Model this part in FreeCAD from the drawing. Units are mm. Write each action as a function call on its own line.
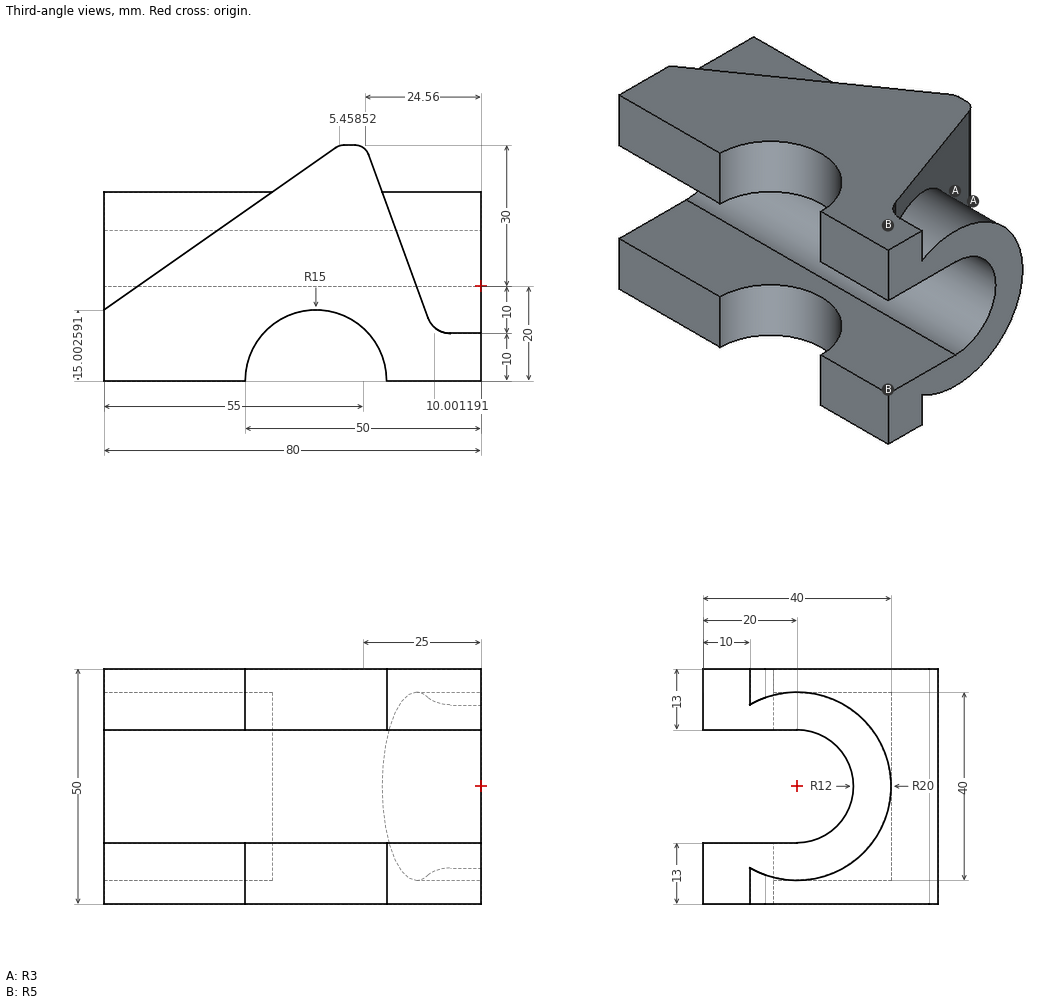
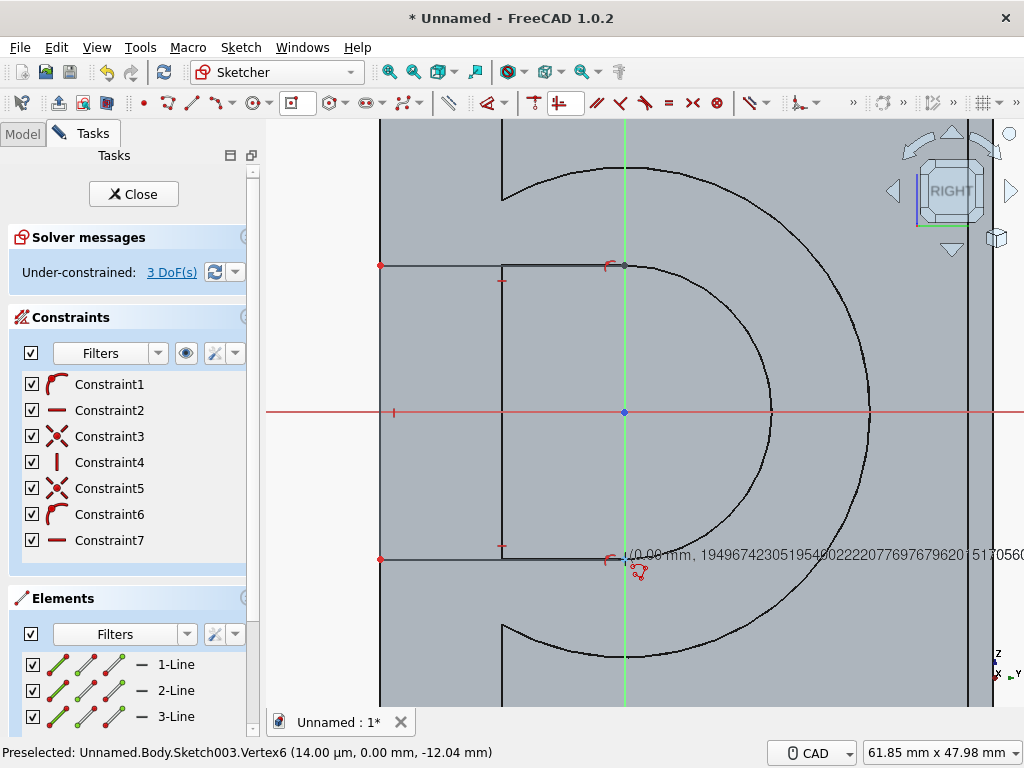
click(216, 104)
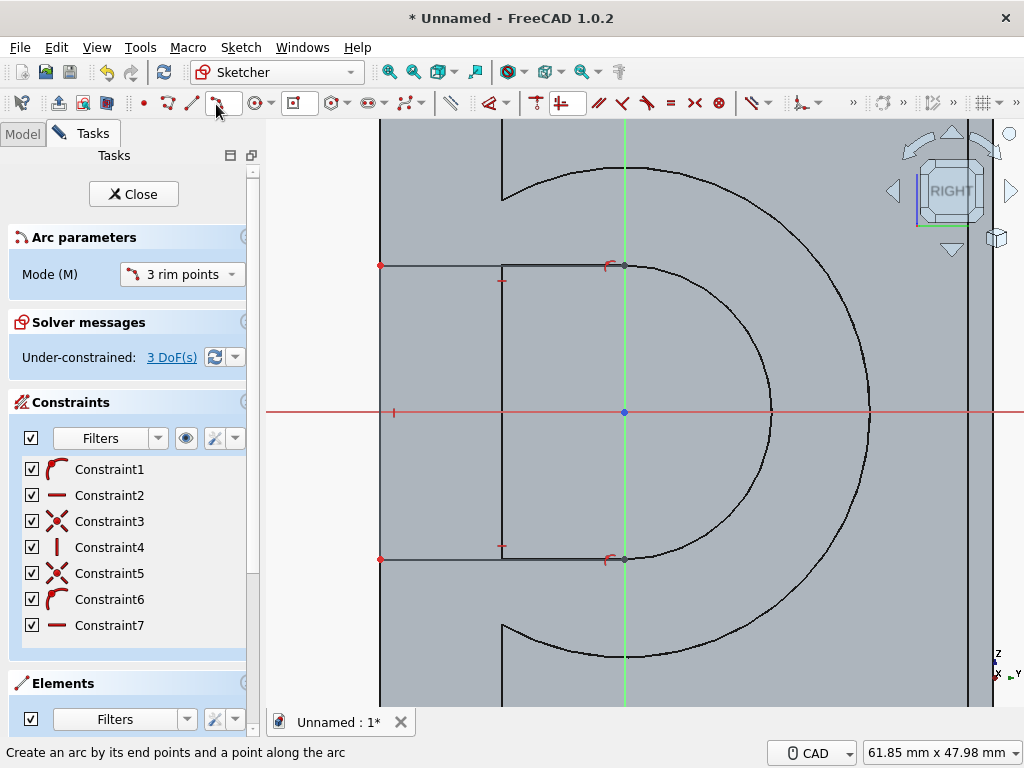
click(625, 560)
click(625, 266)
click(765, 458)
key(Escape)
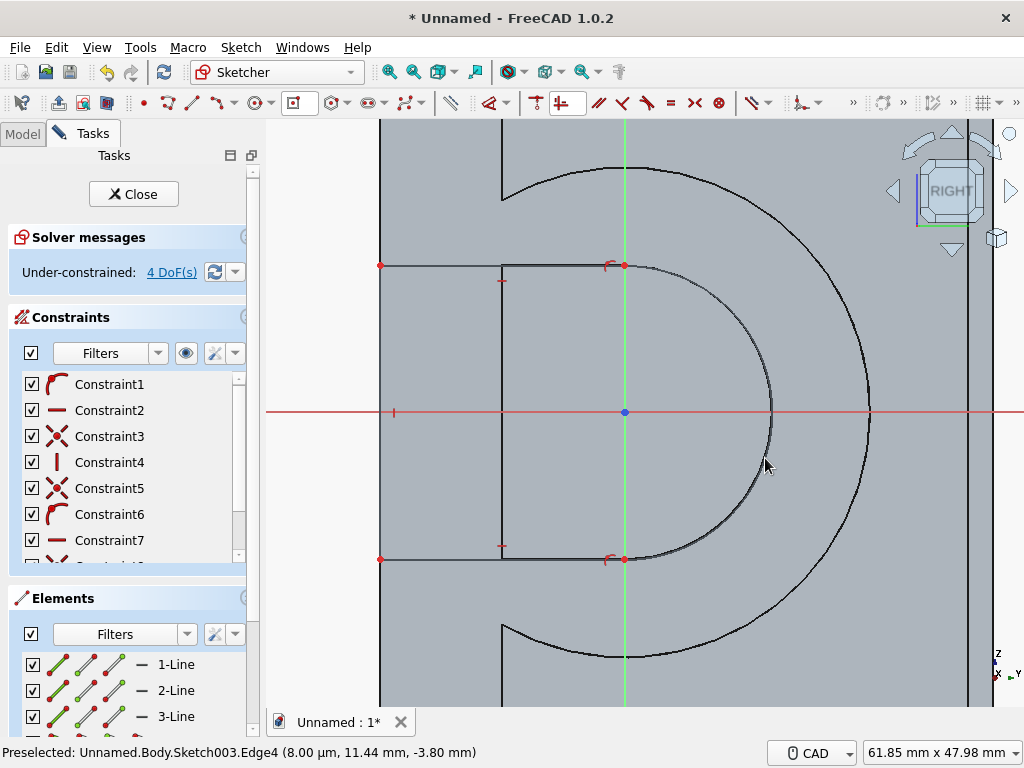
click(551, 266)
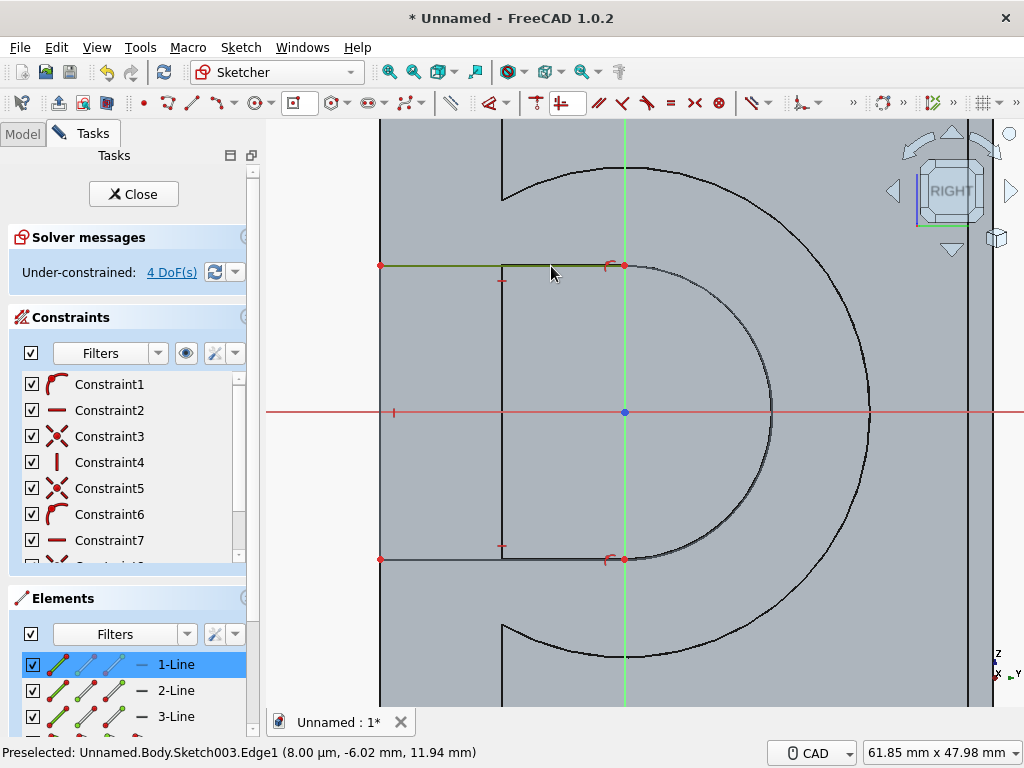
click(744, 500)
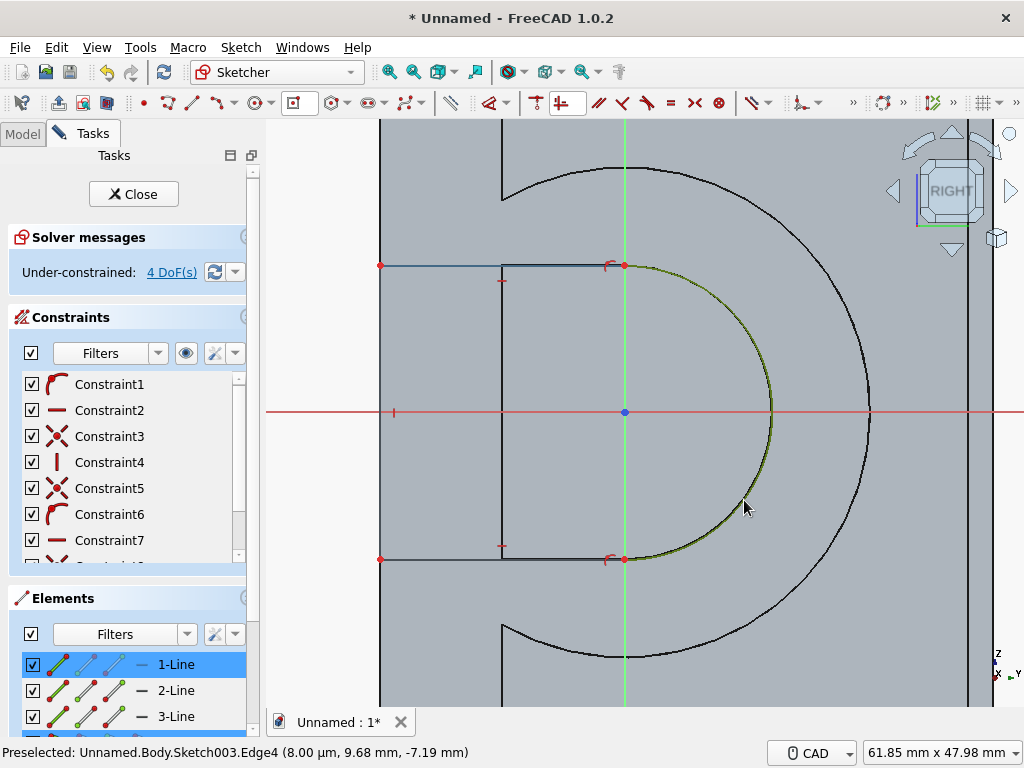
click(648, 104)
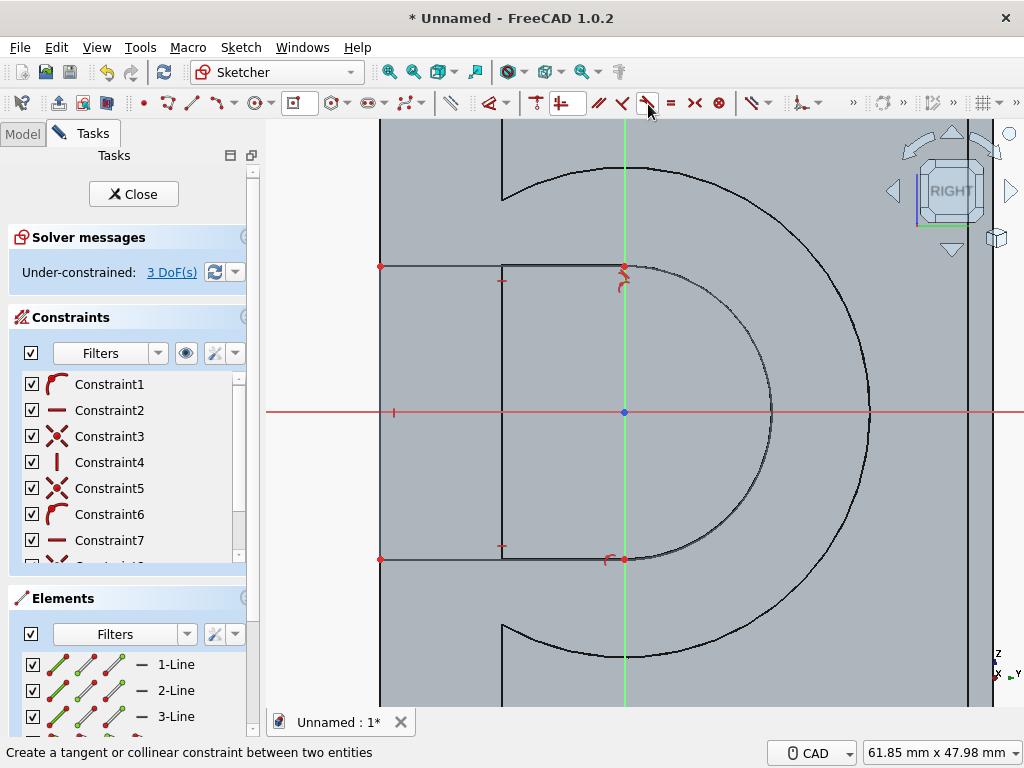
click(625, 413)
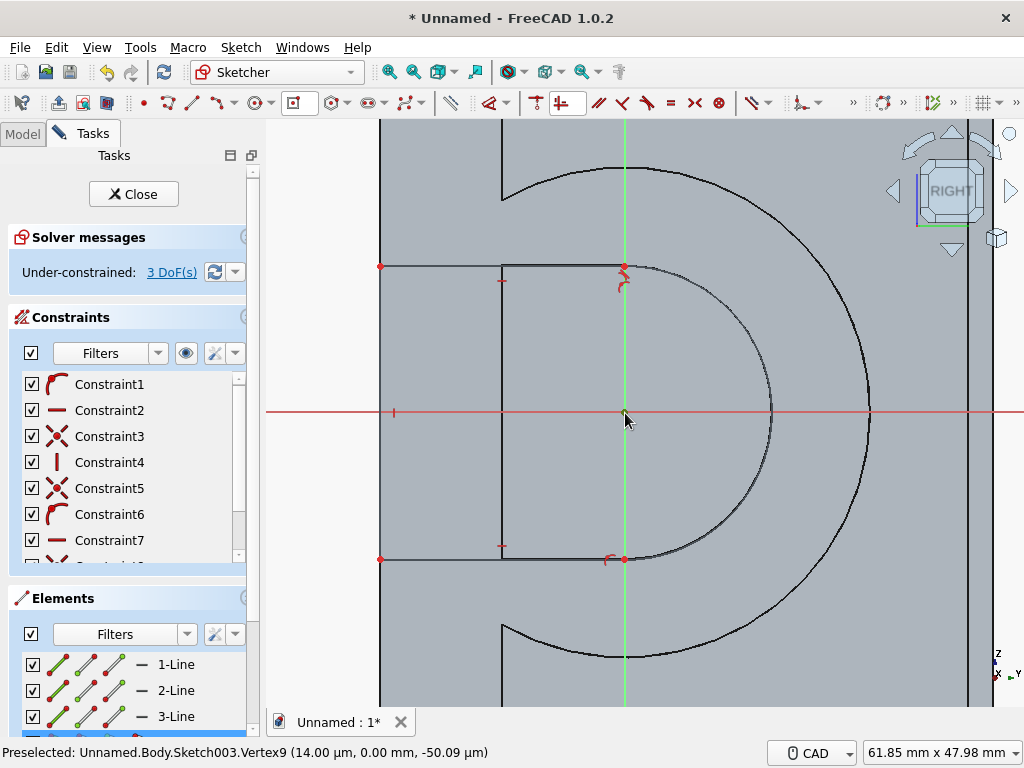
click(334, 412)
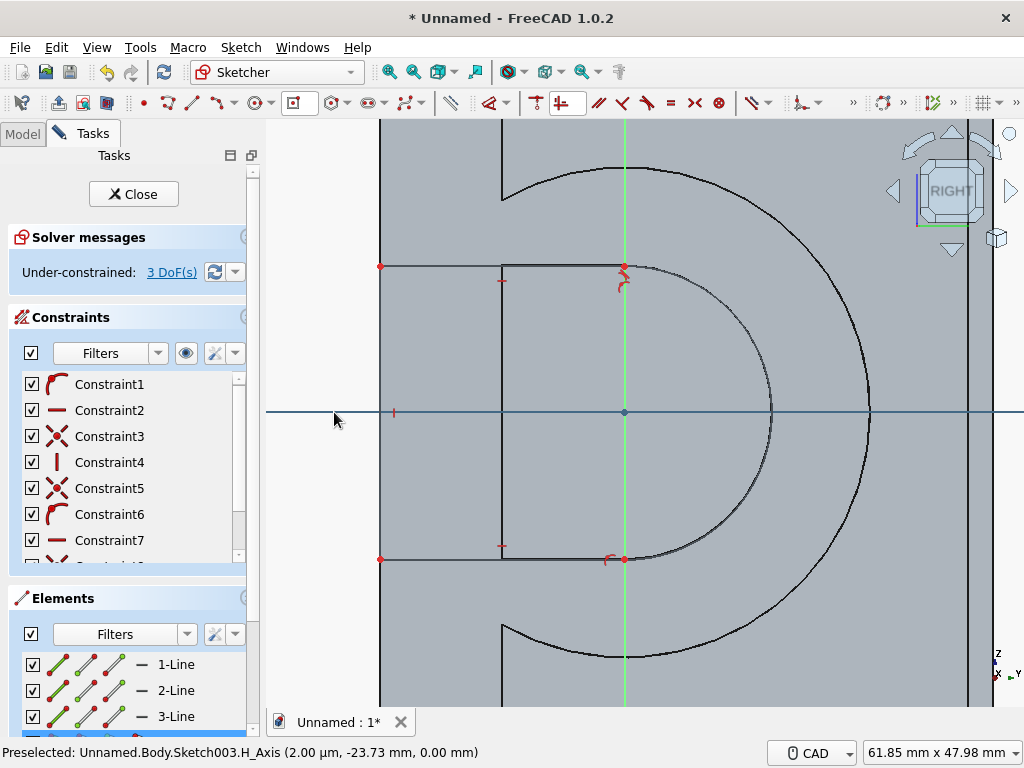
click(536, 104)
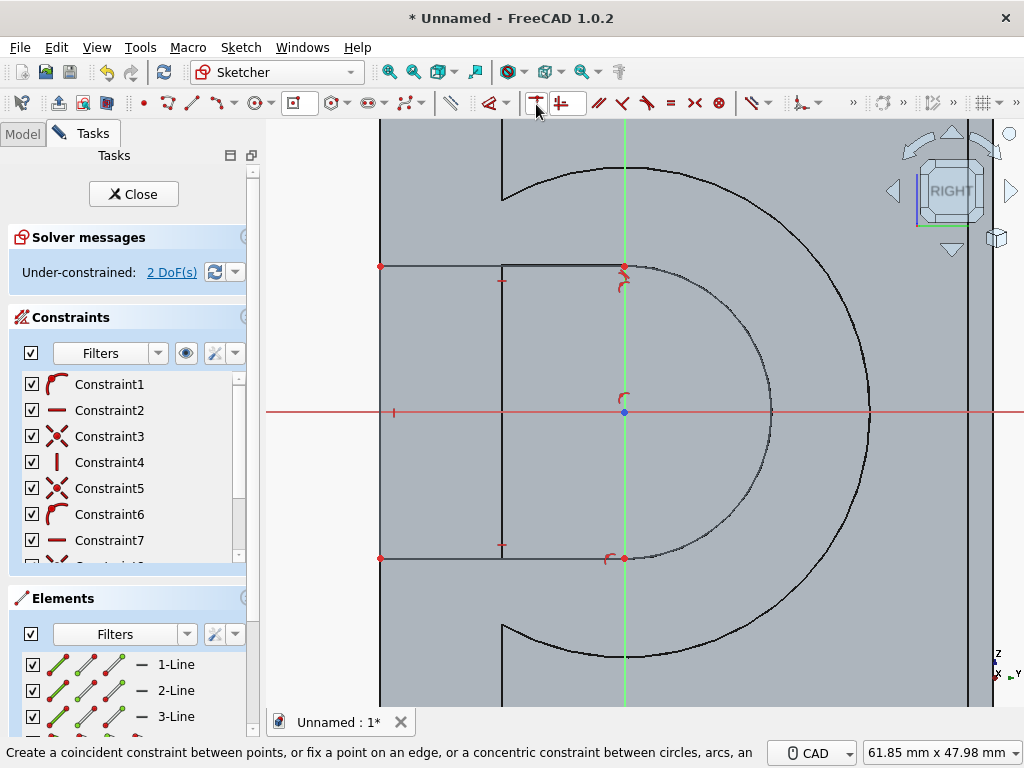
click(490, 104)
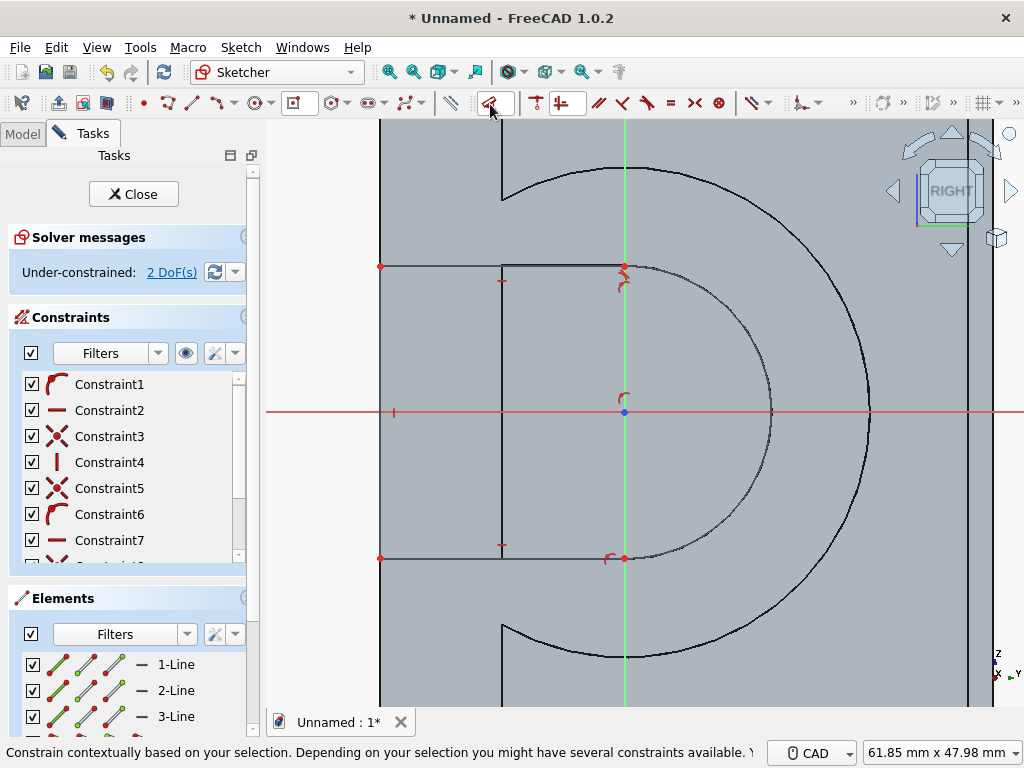
click(743, 498)
click(769, 517)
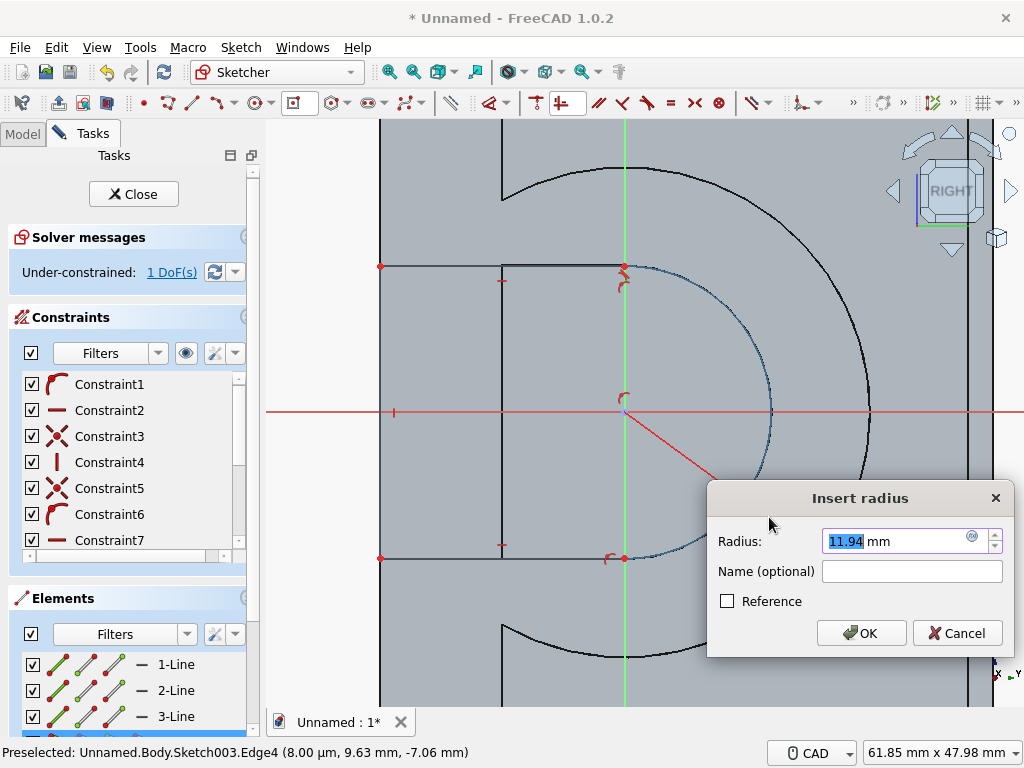
text(12)
key(Return)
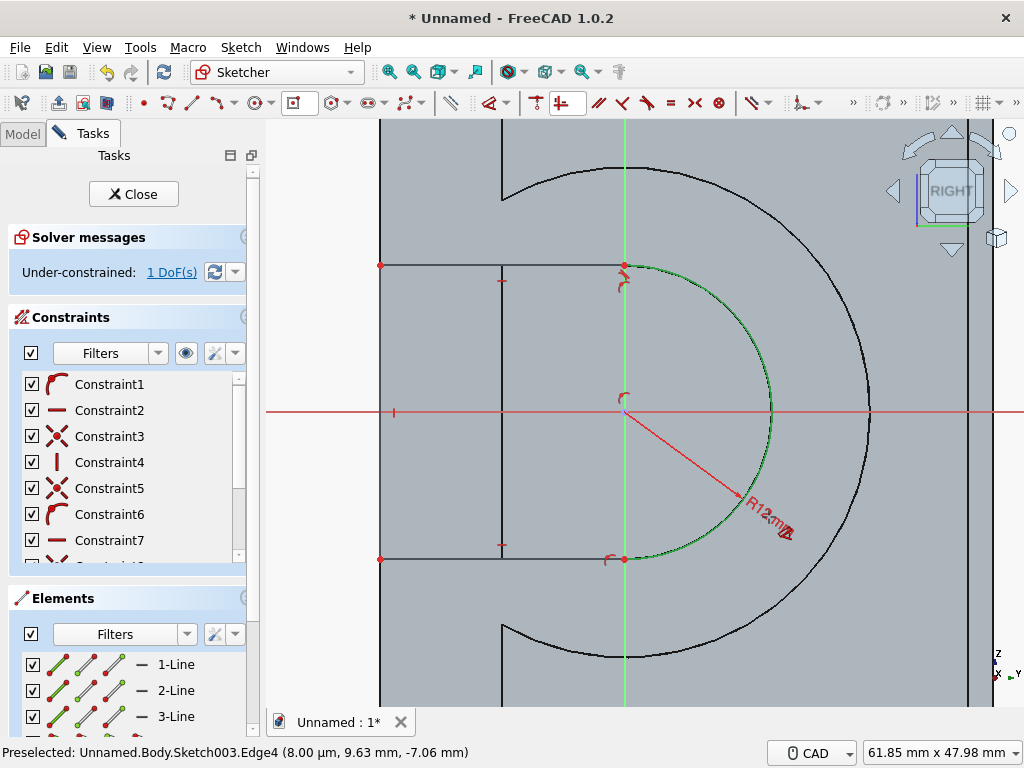
click(551, 265)
click(502, 231)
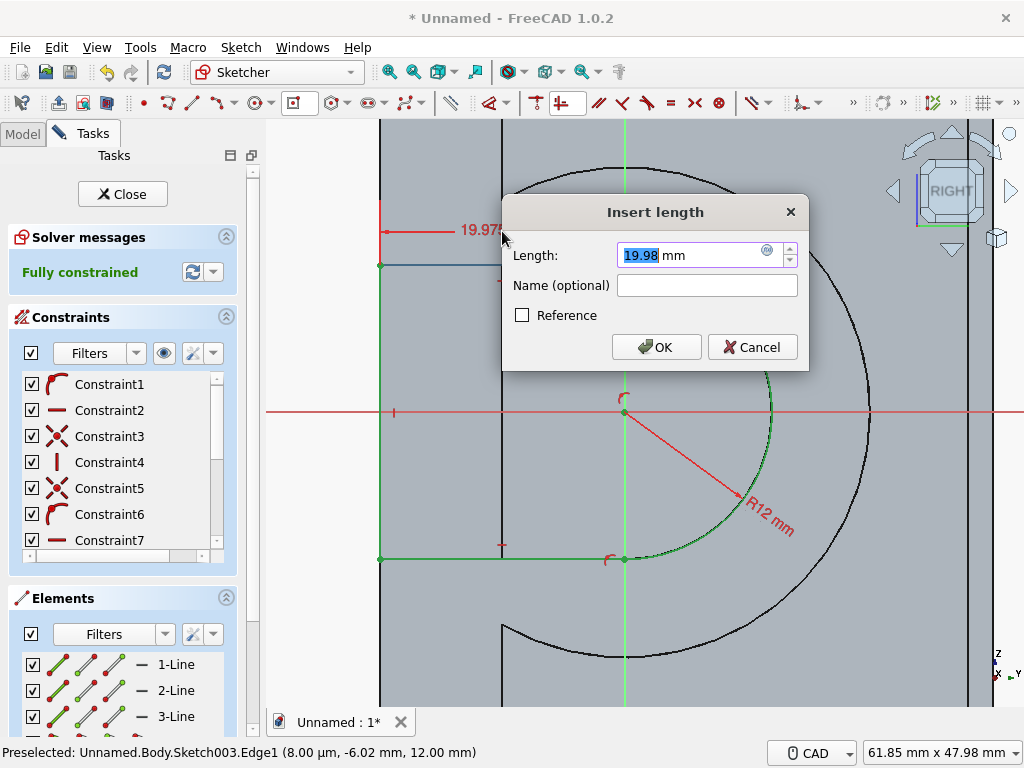
text(20)
key(Return)
key(Escape)